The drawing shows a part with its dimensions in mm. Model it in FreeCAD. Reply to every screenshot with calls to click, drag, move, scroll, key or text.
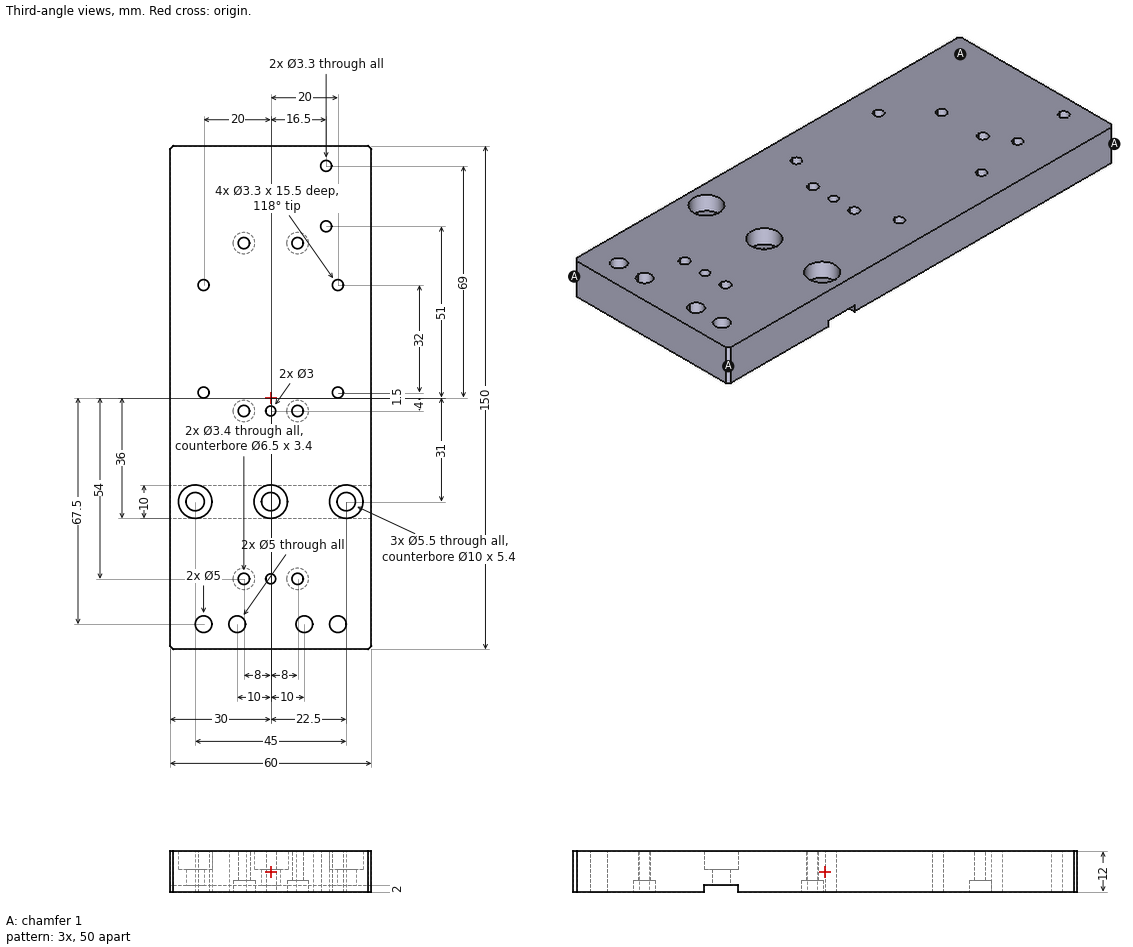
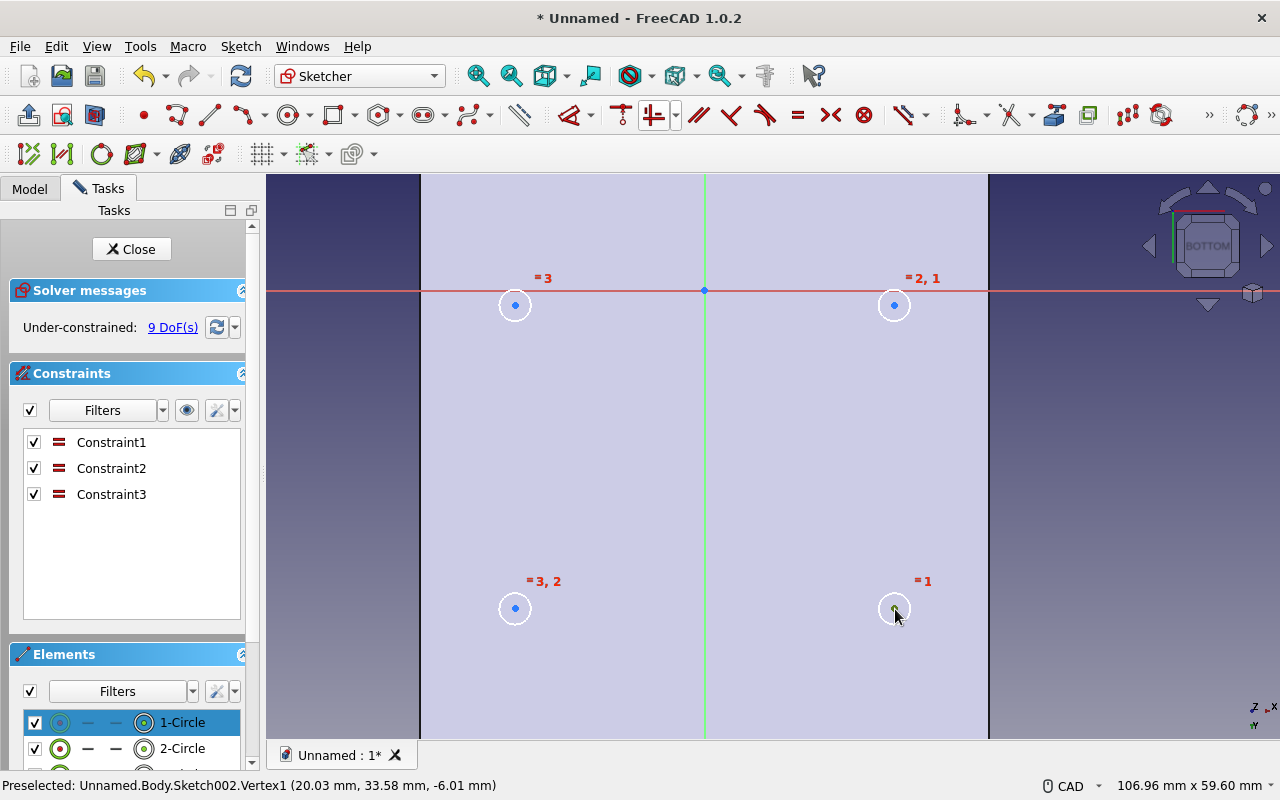
click(894, 305)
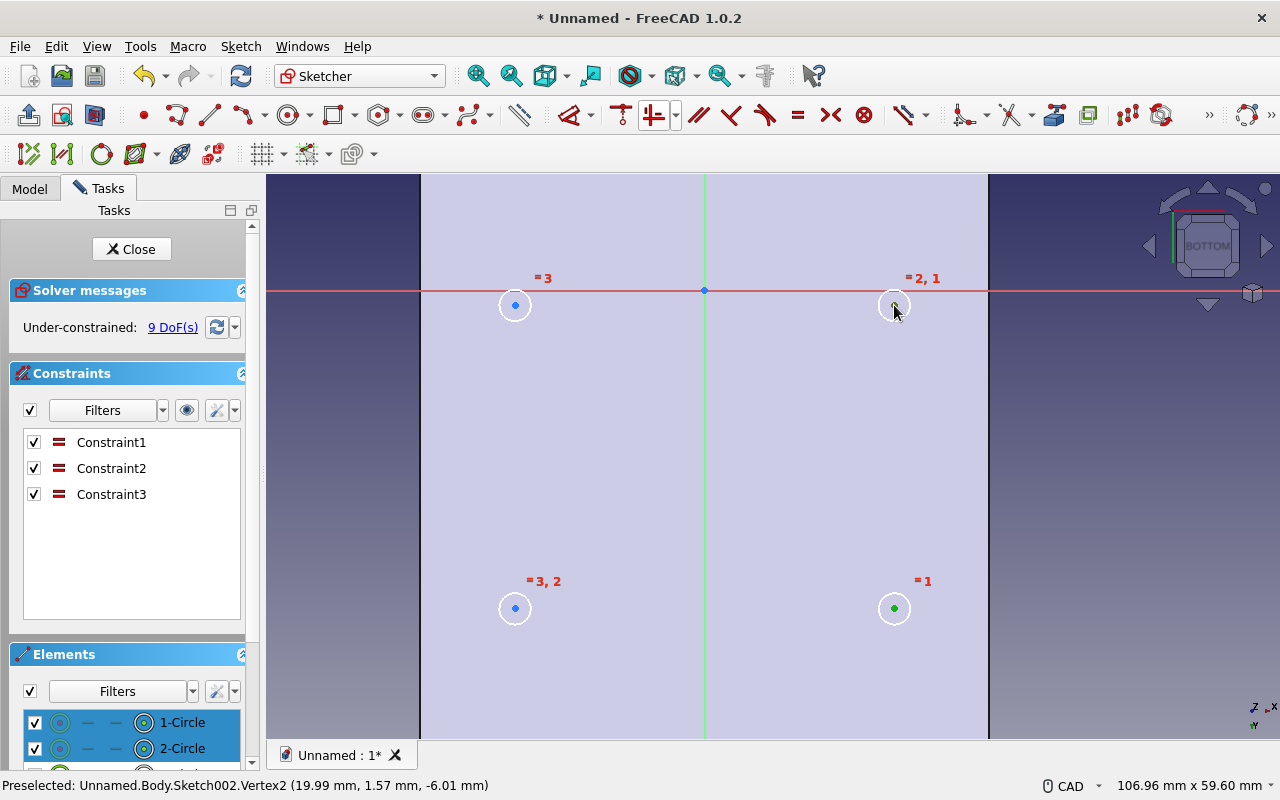
key(v)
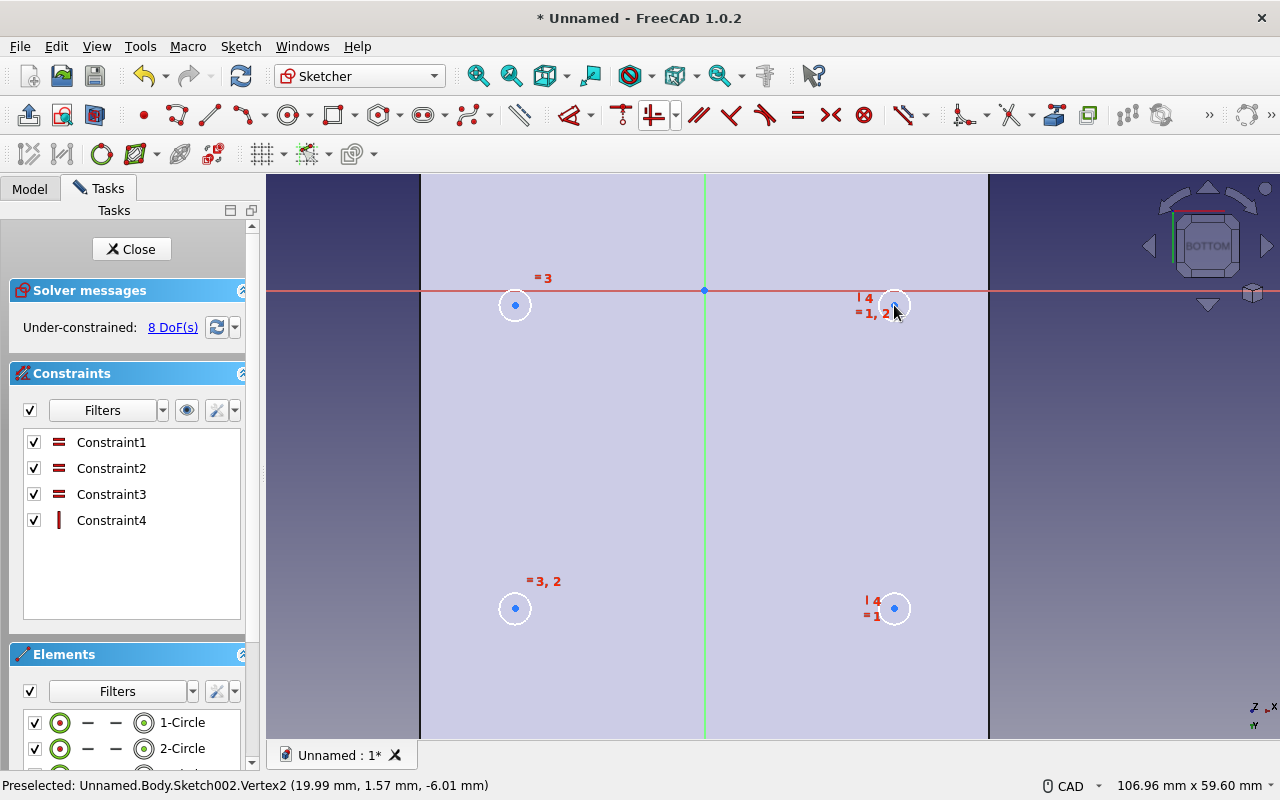
click(895, 609)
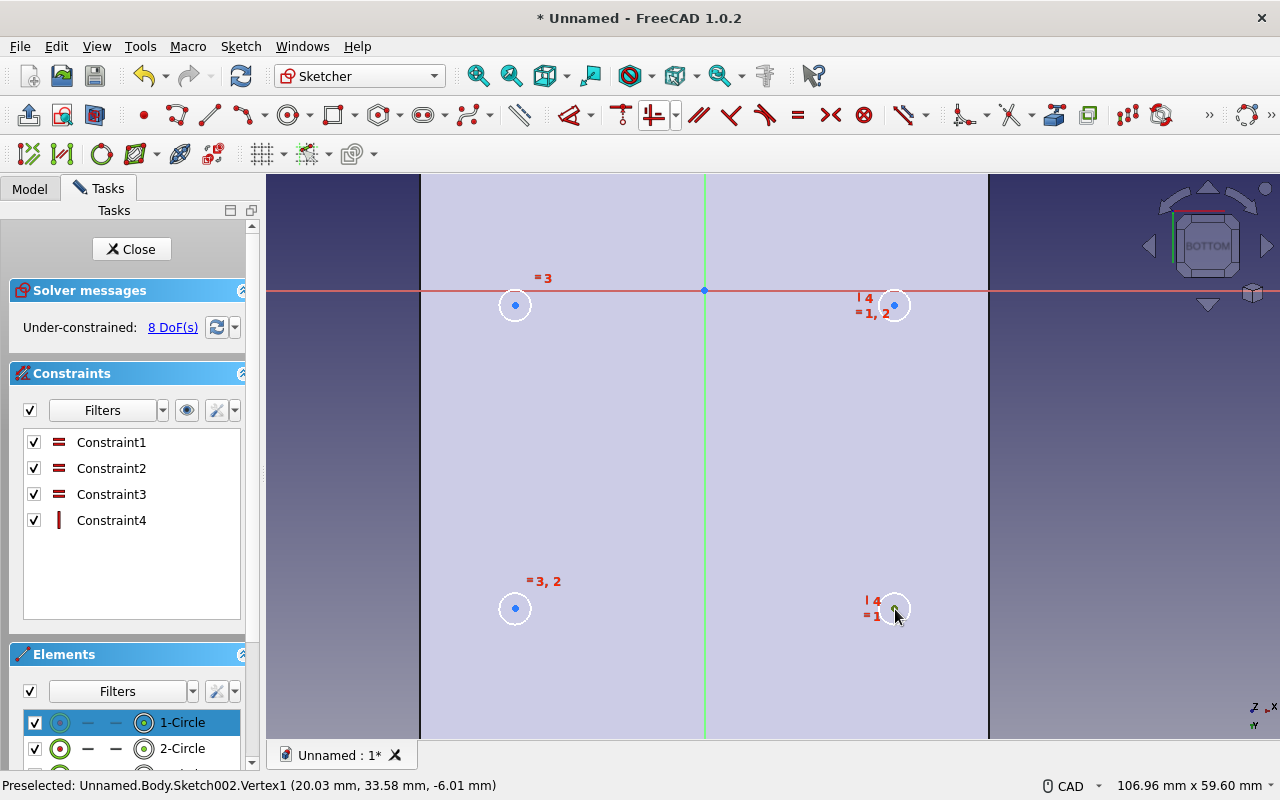
click(515, 609)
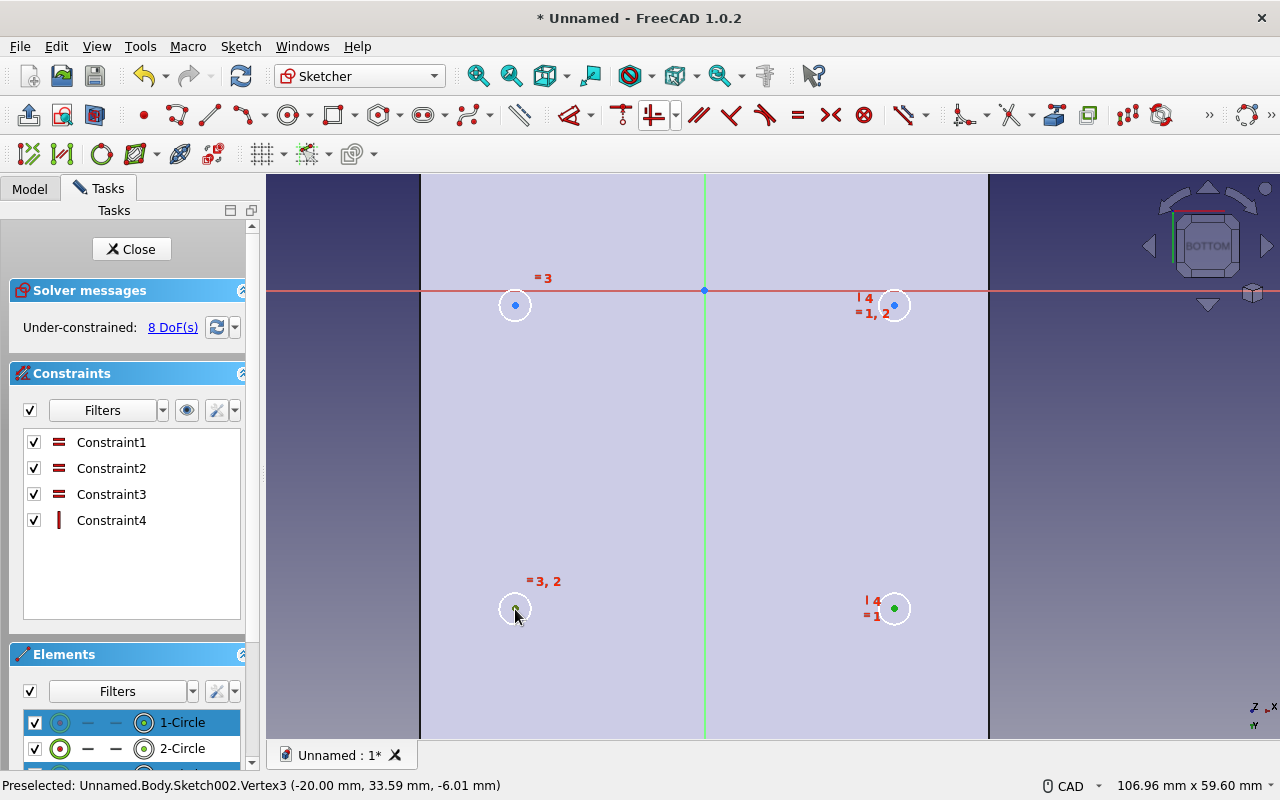
click(676, 116)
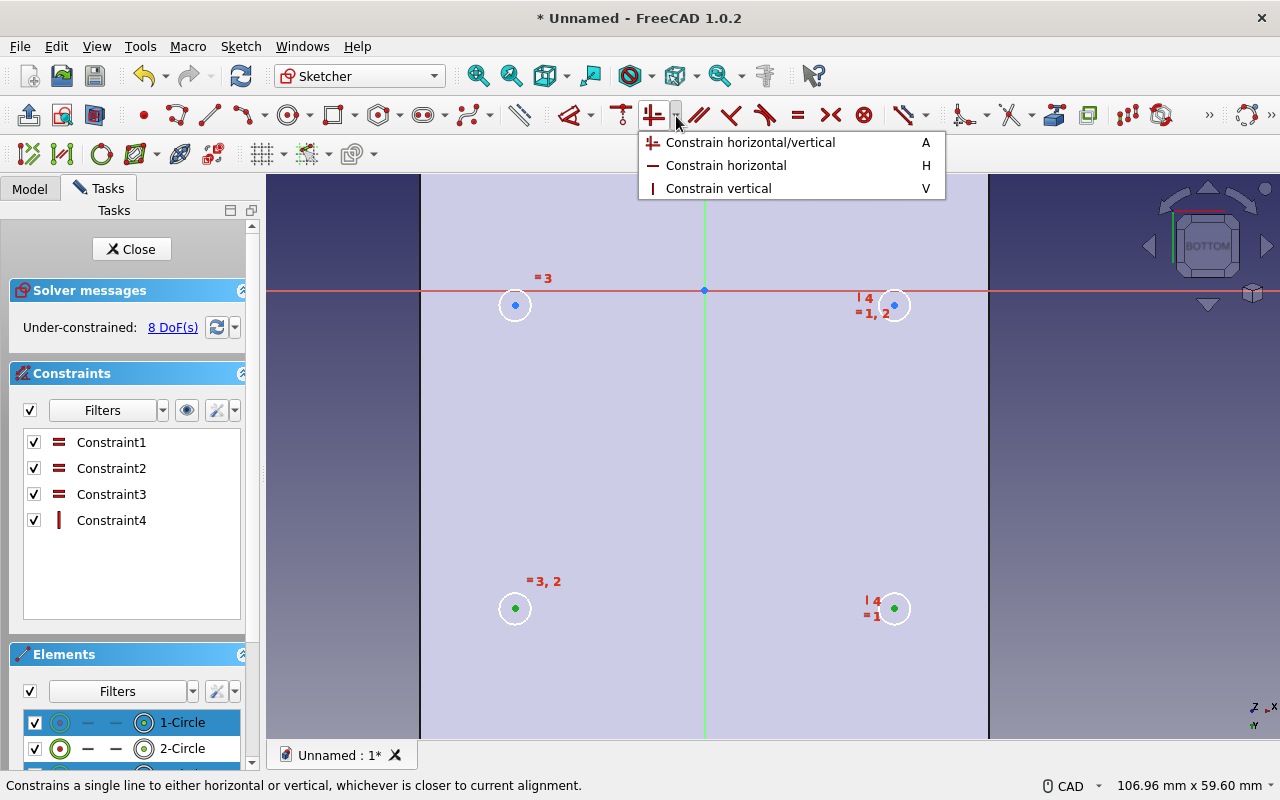
click(792, 166)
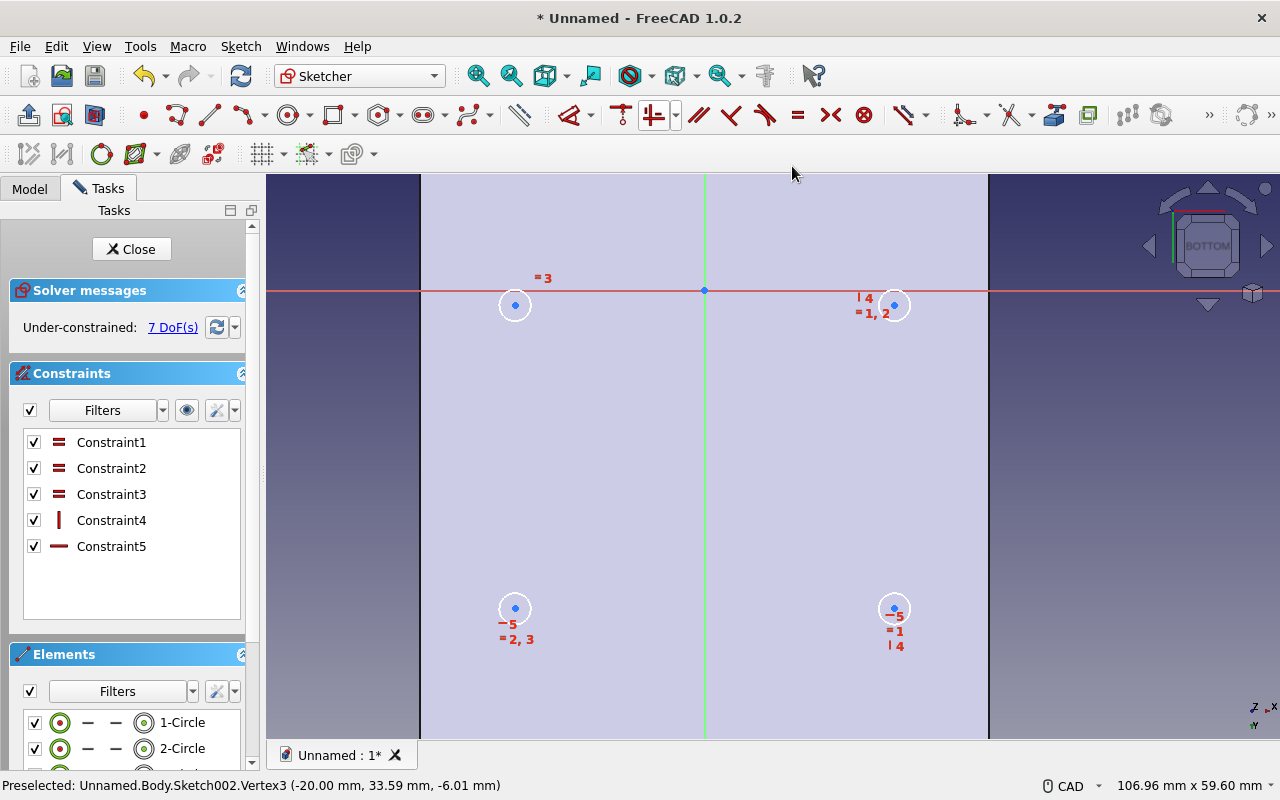
click(515, 609)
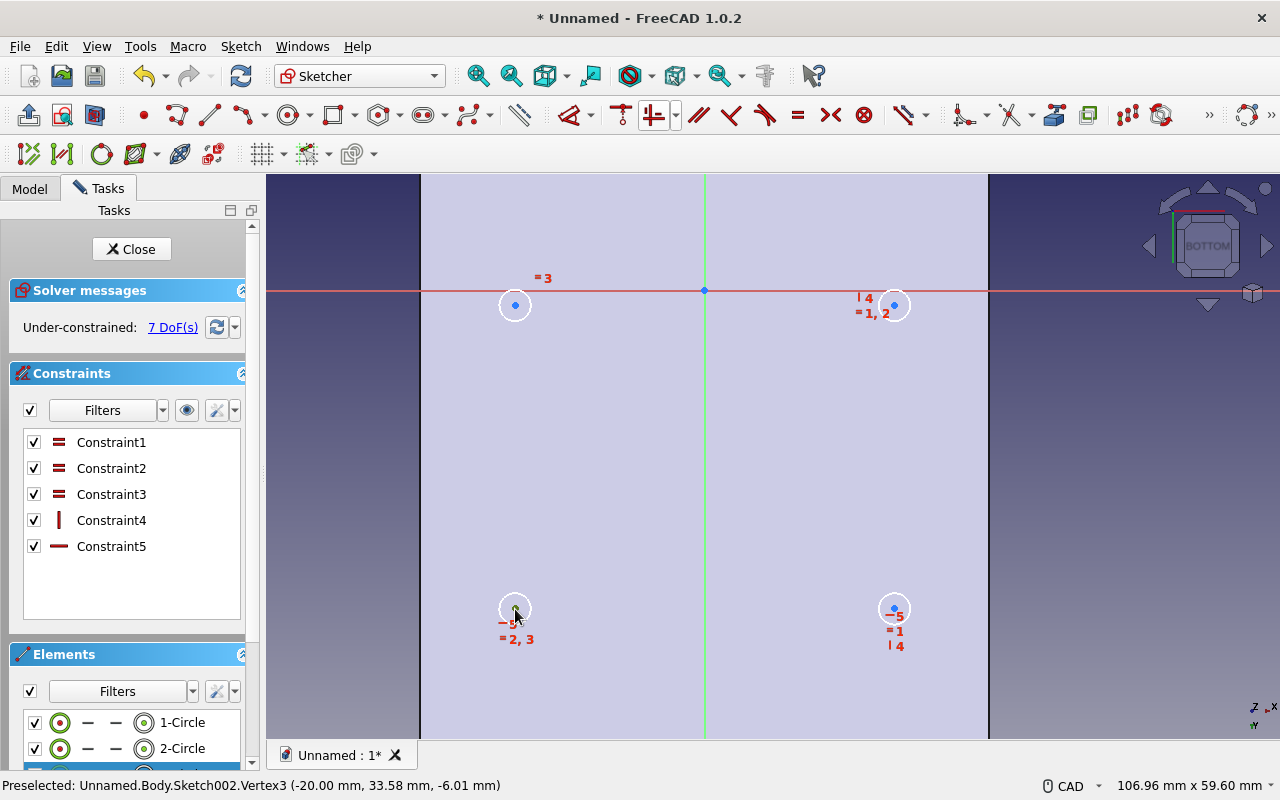
click(515, 305)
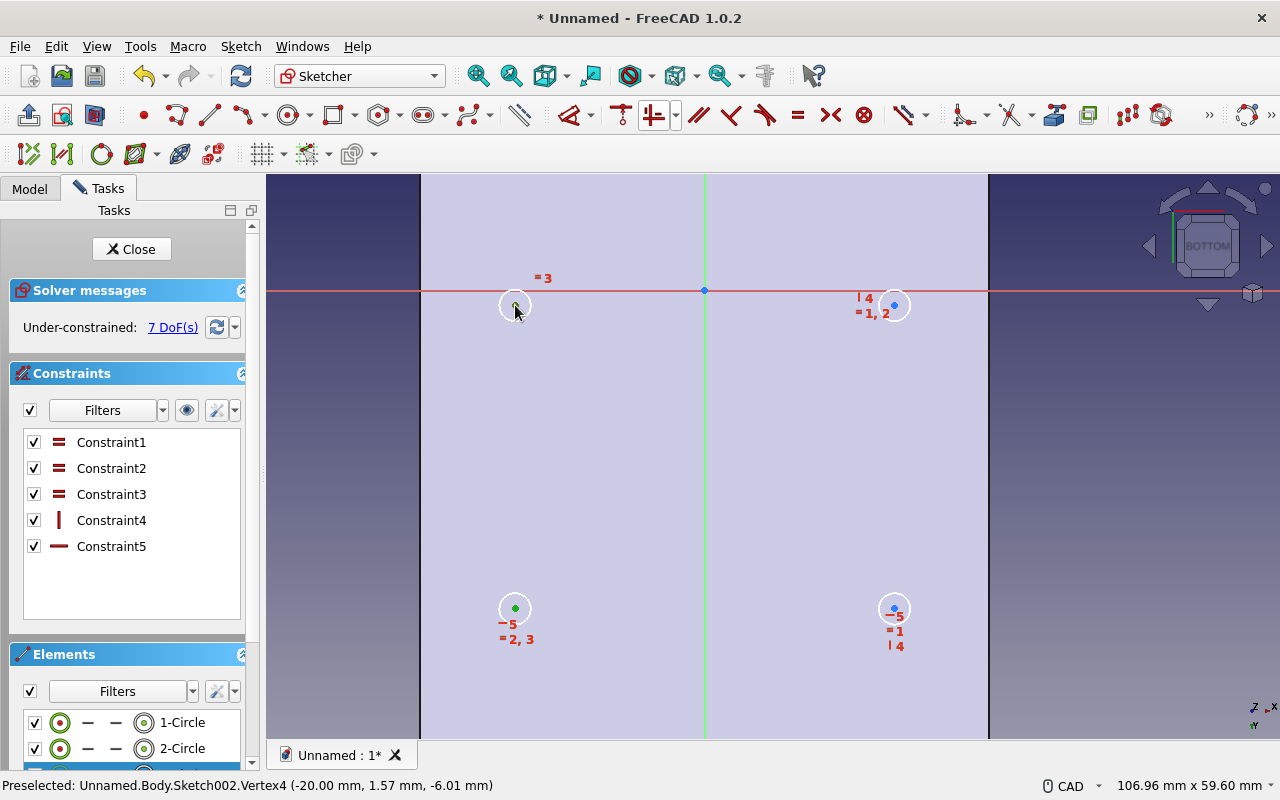
click(676, 116)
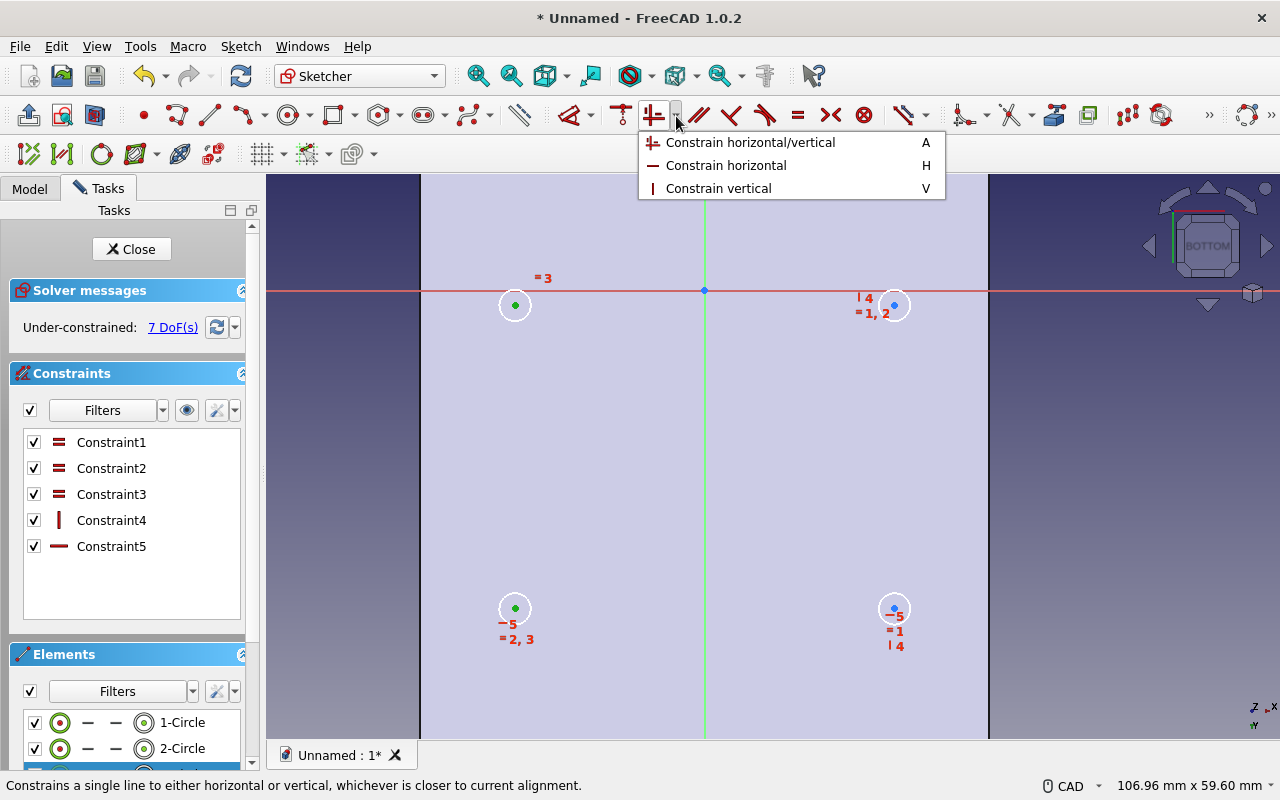
click(792, 188)